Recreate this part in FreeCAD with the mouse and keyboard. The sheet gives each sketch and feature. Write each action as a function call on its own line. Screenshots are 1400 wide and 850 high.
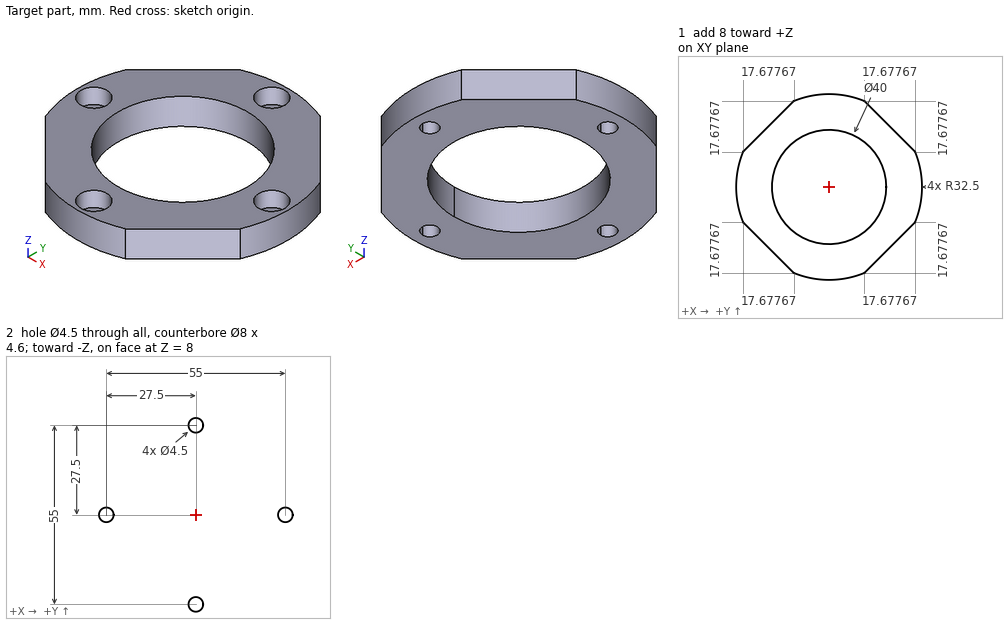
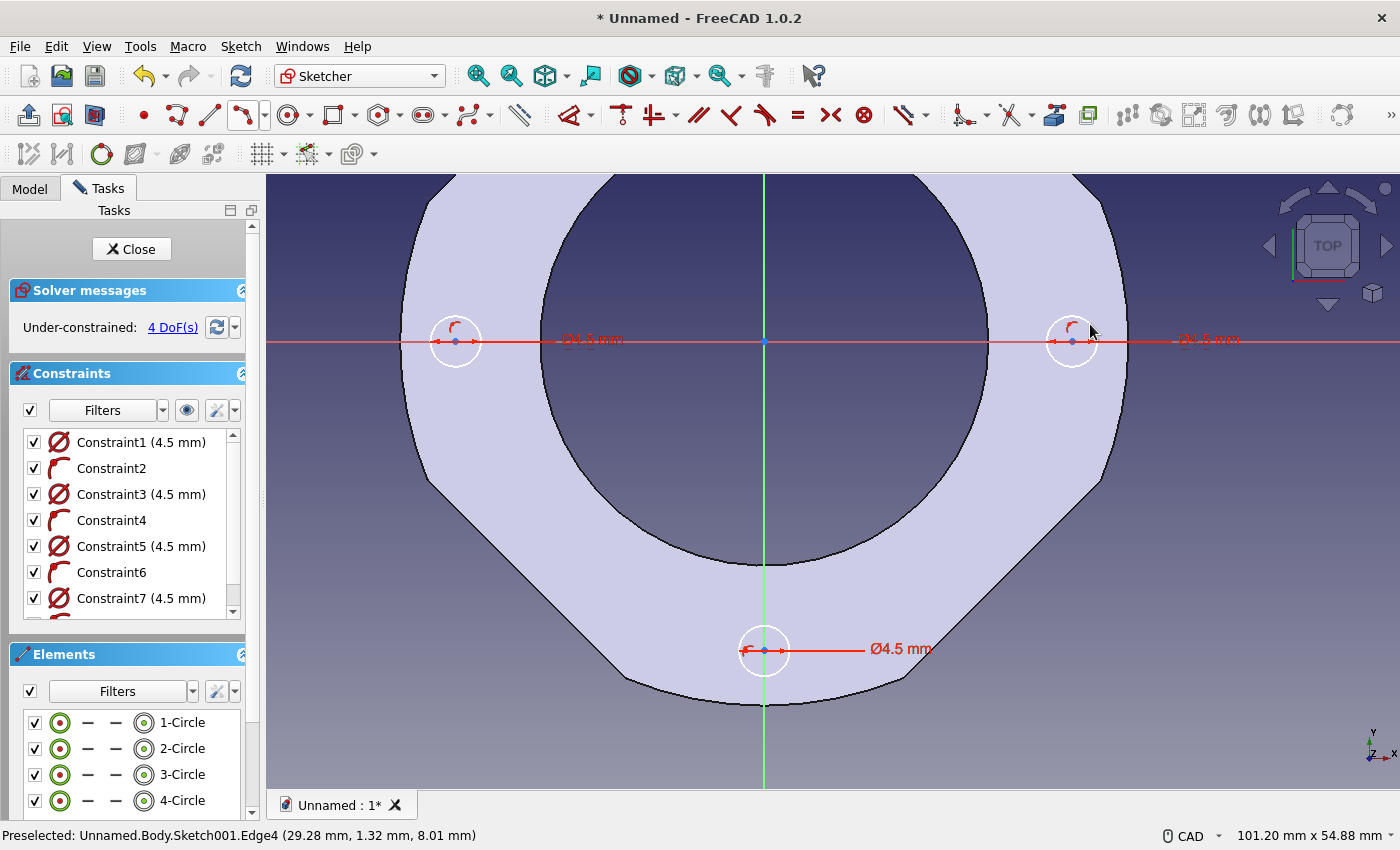
click(568, 116)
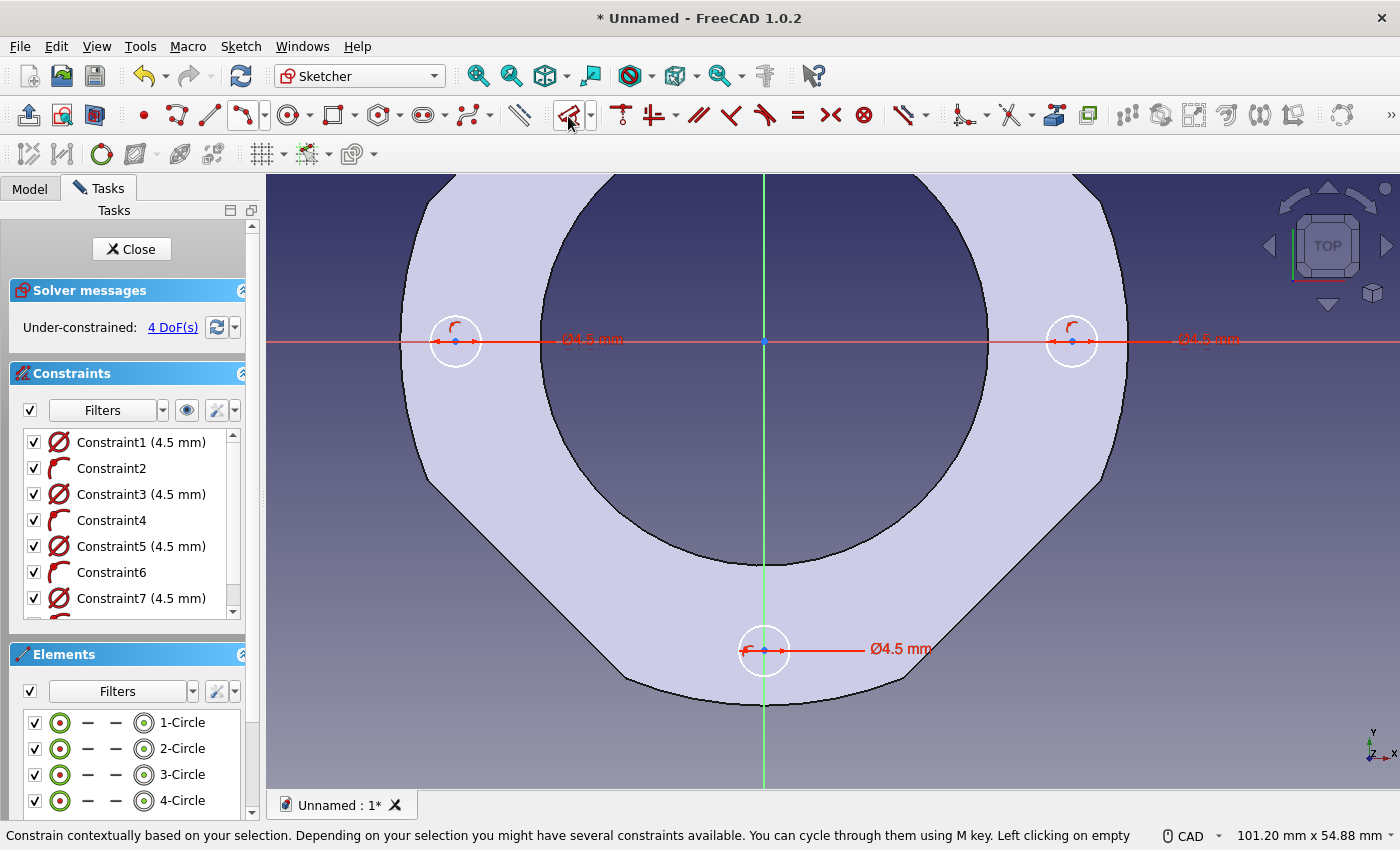
scroll(765, 652, down, 3)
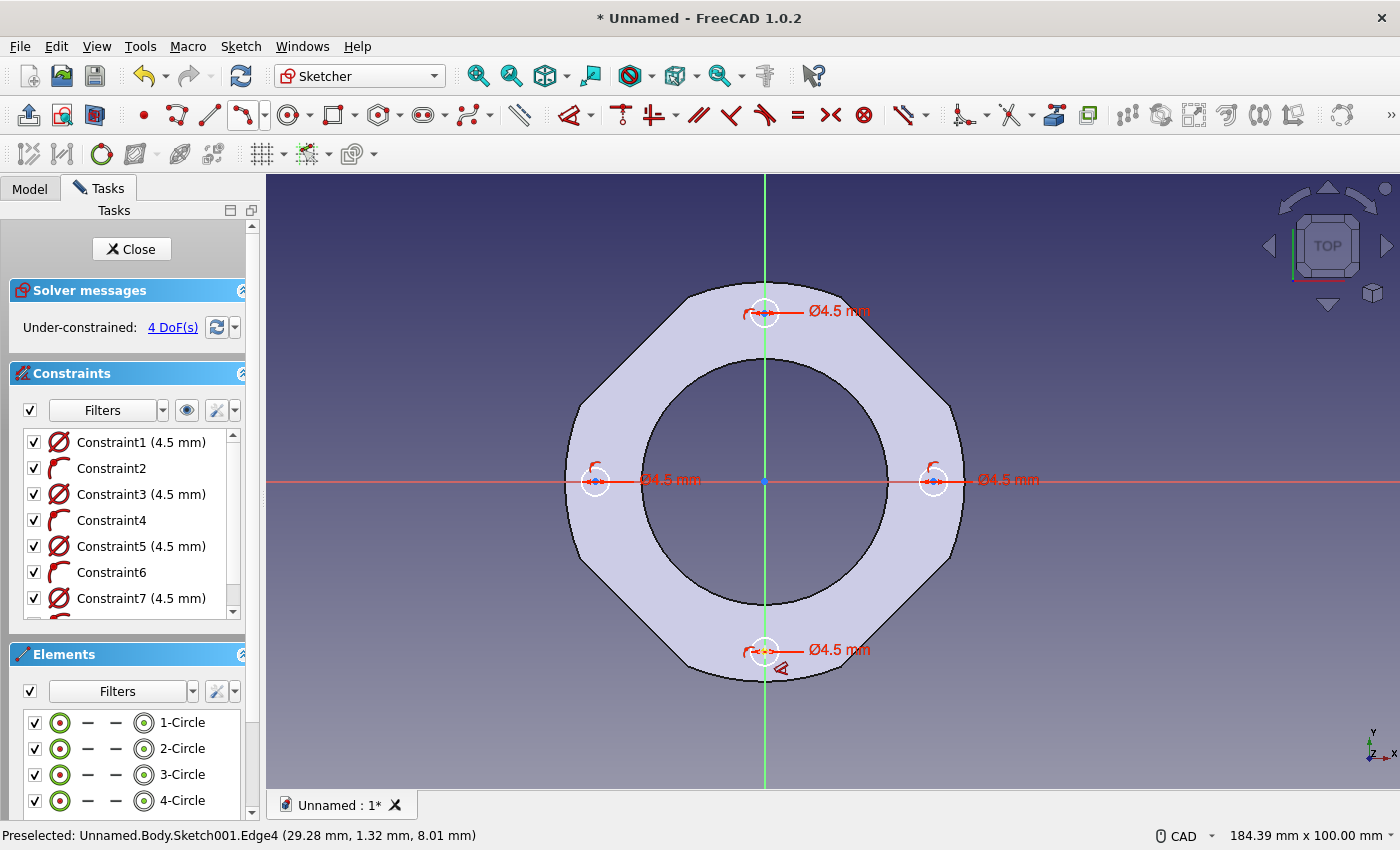
click(765, 313)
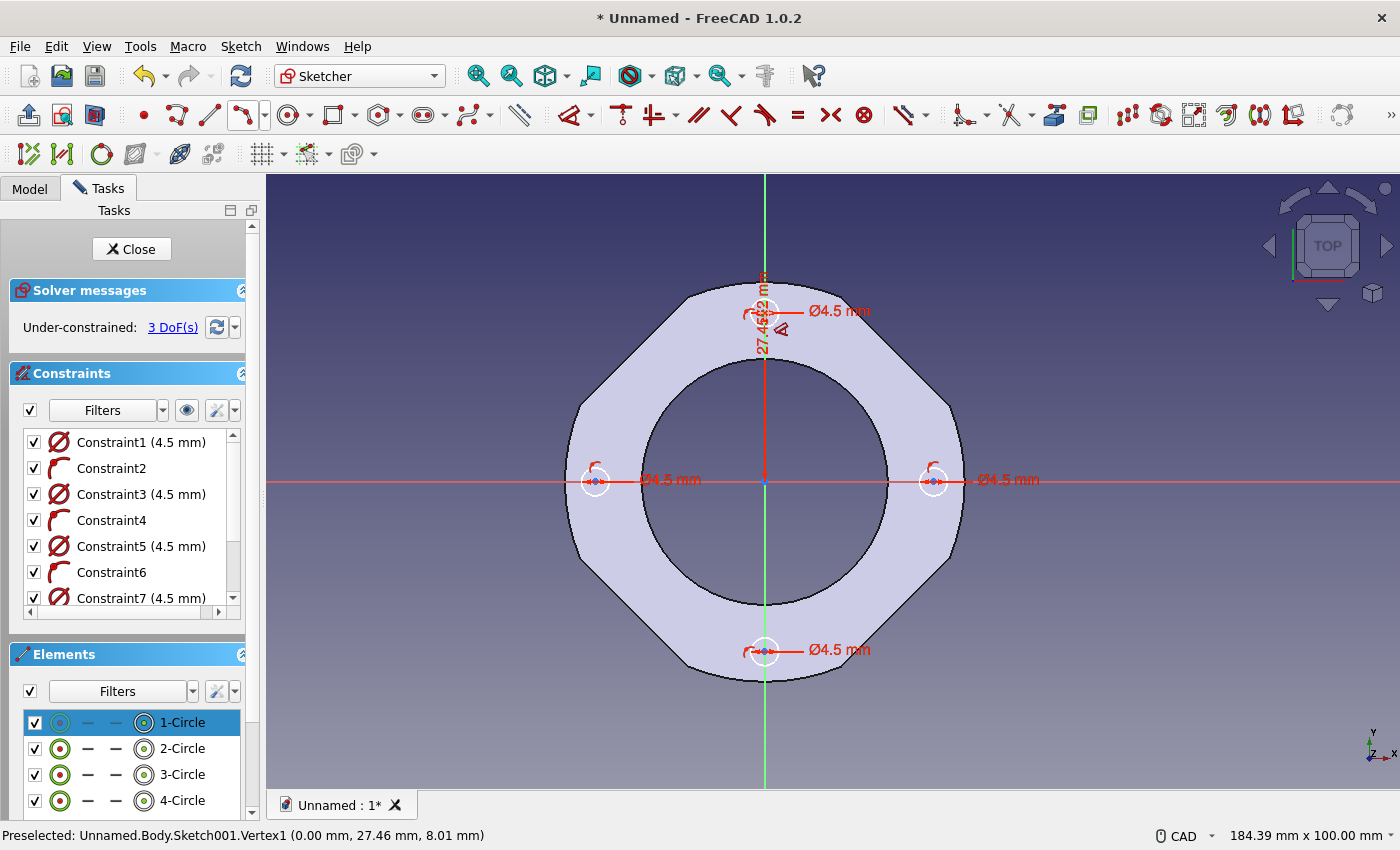
click(765, 652)
click(799, 405)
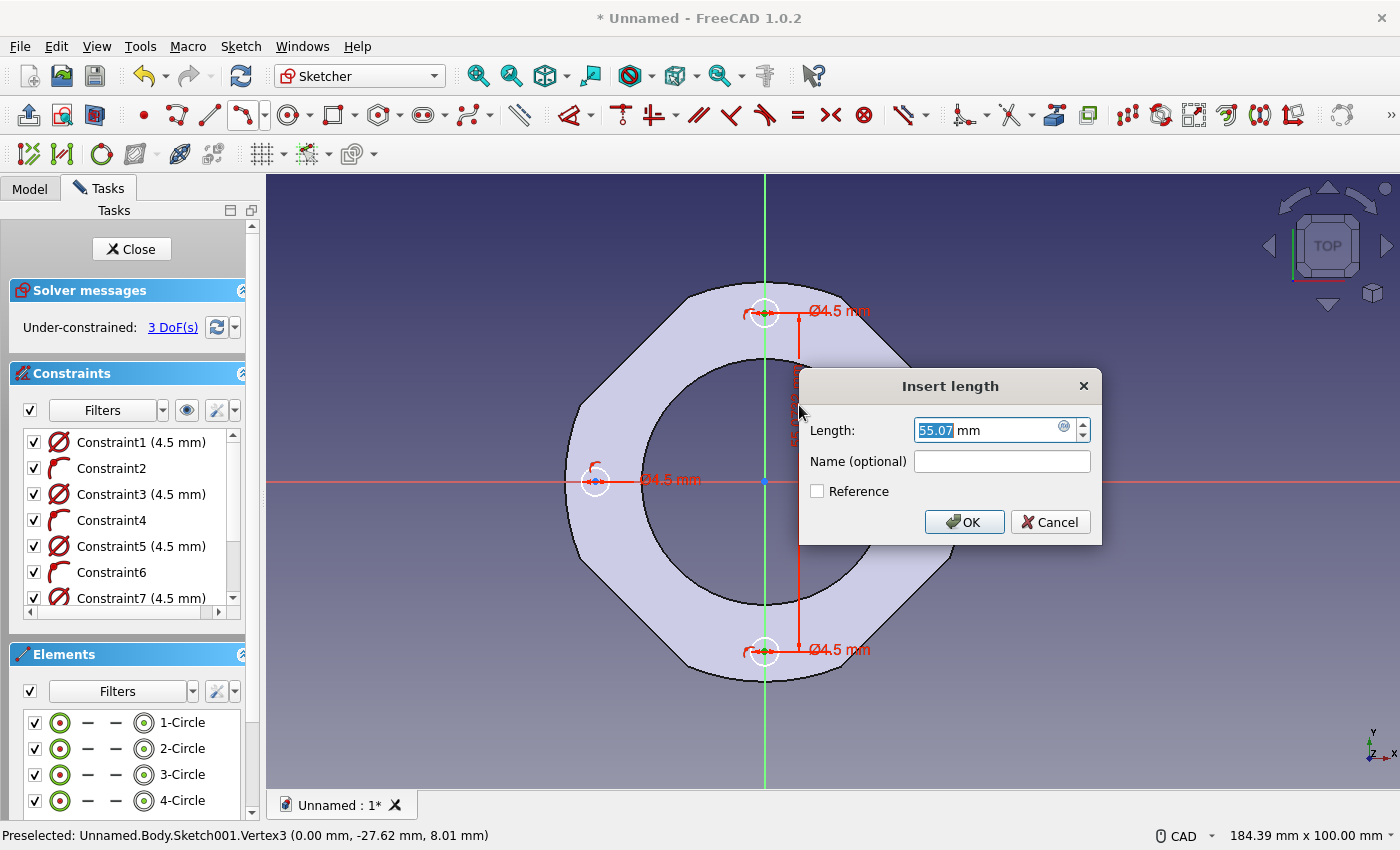
text(55)
key(Return)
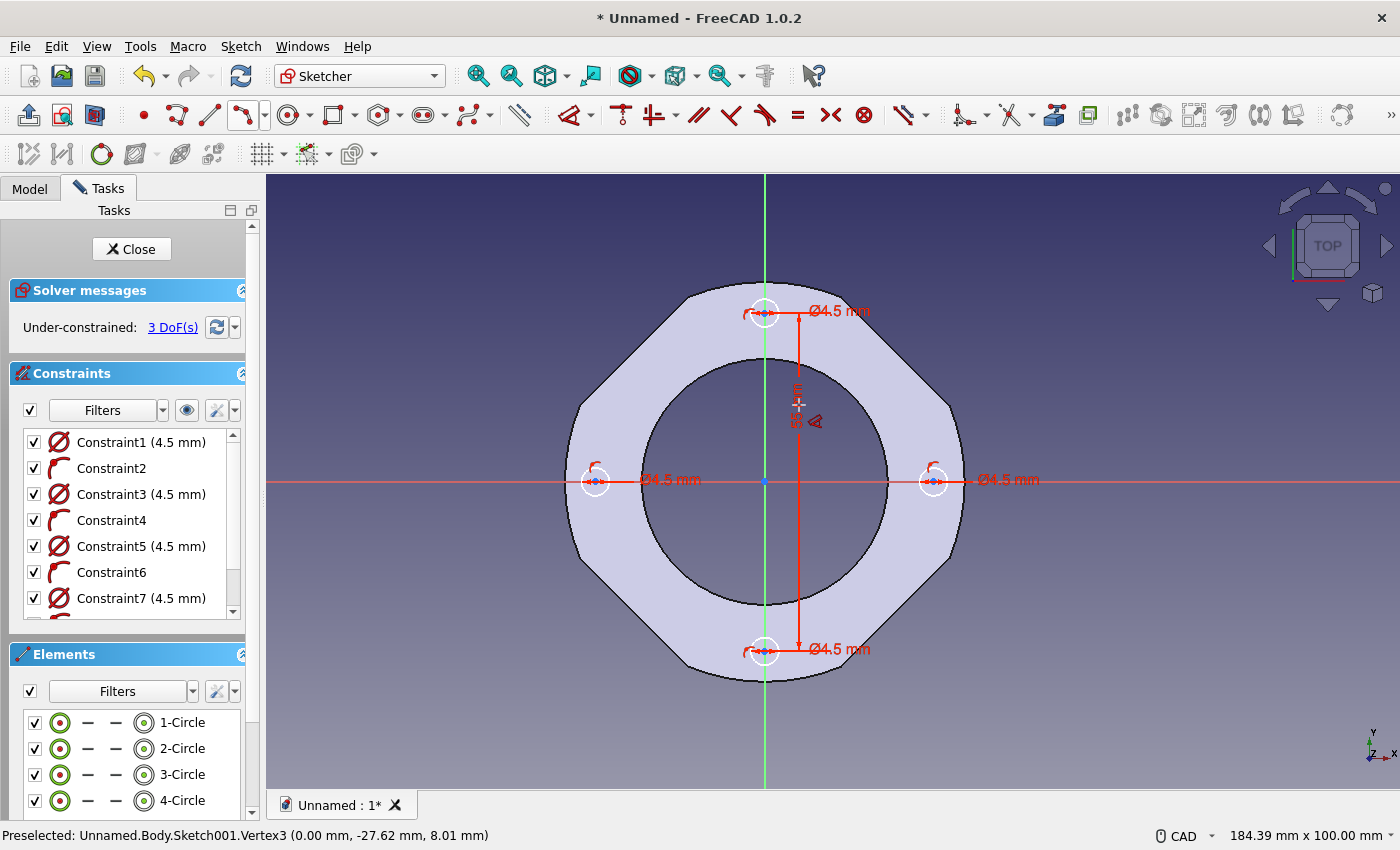
click(595, 482)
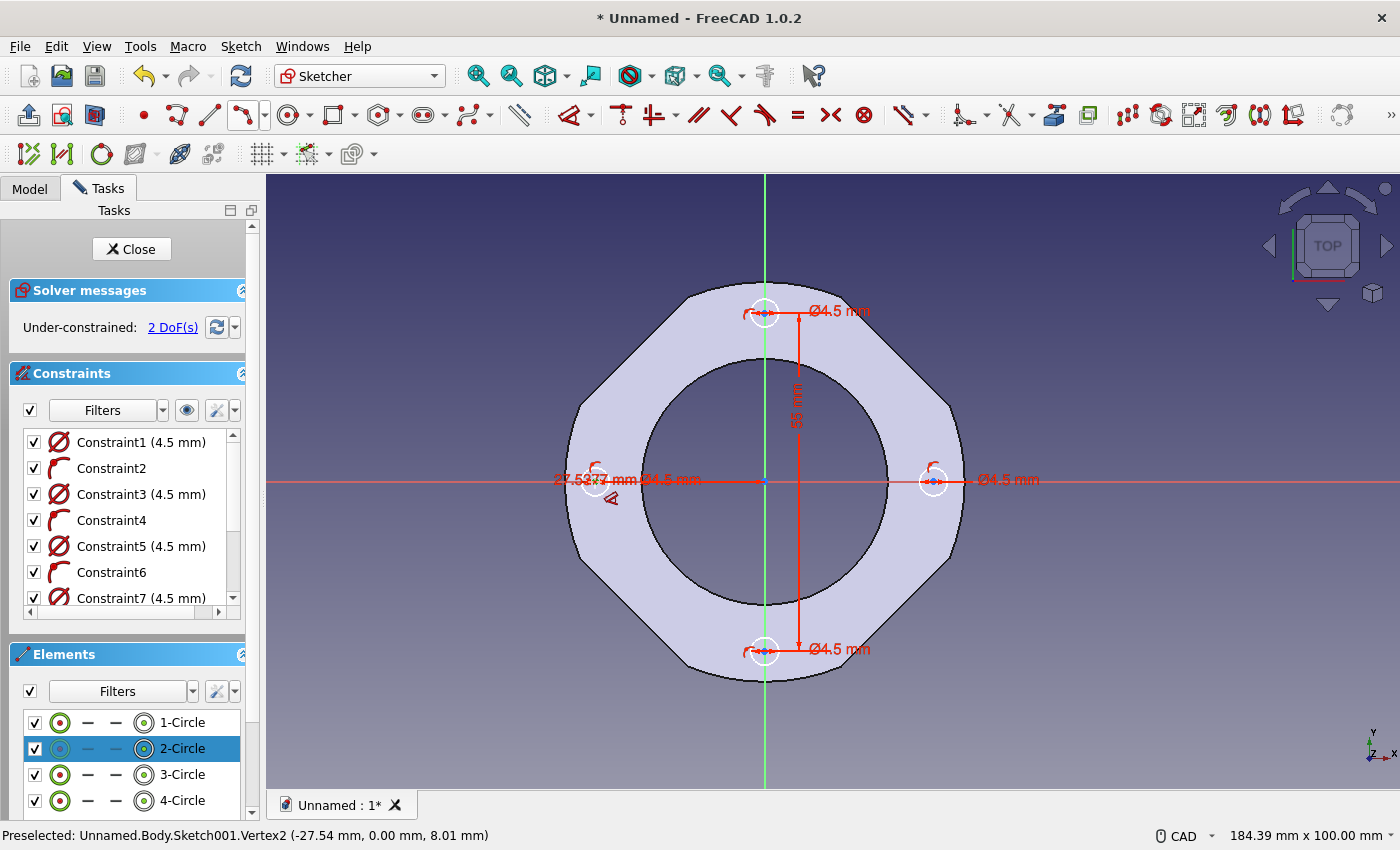
click(934, 482)
click(687, 516)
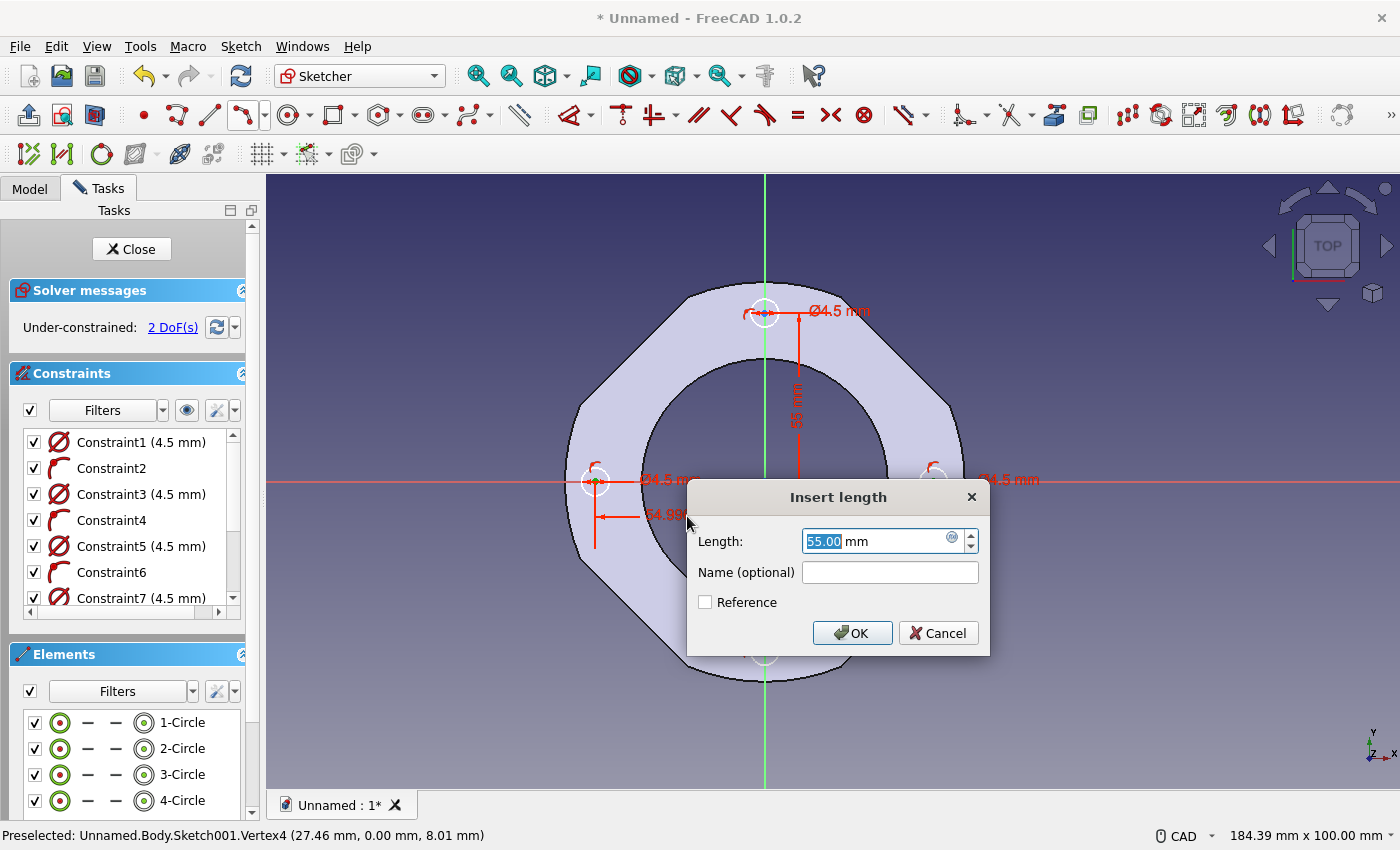
text(55)
key(Return)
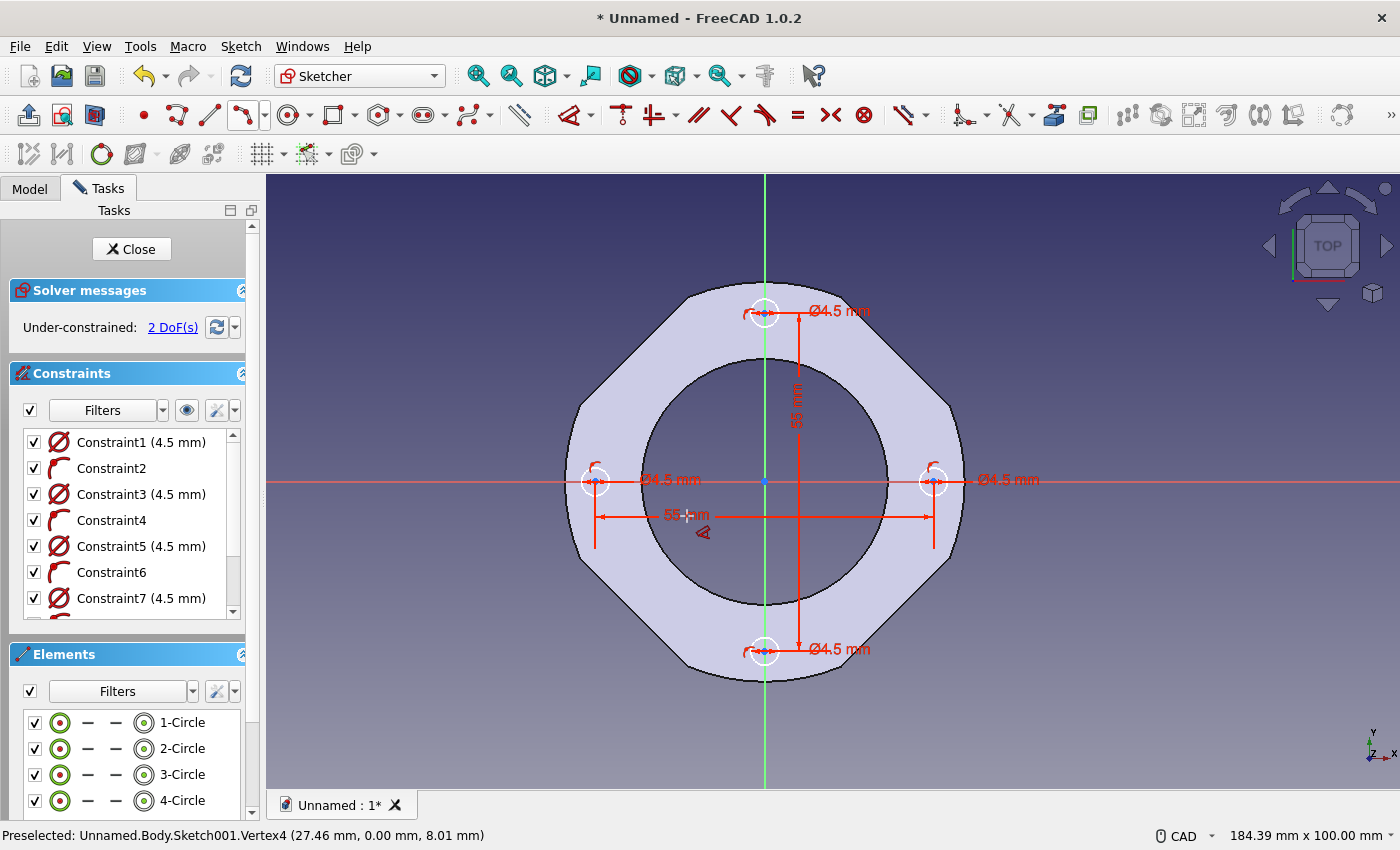
click(765, 313)
click(799, 359)